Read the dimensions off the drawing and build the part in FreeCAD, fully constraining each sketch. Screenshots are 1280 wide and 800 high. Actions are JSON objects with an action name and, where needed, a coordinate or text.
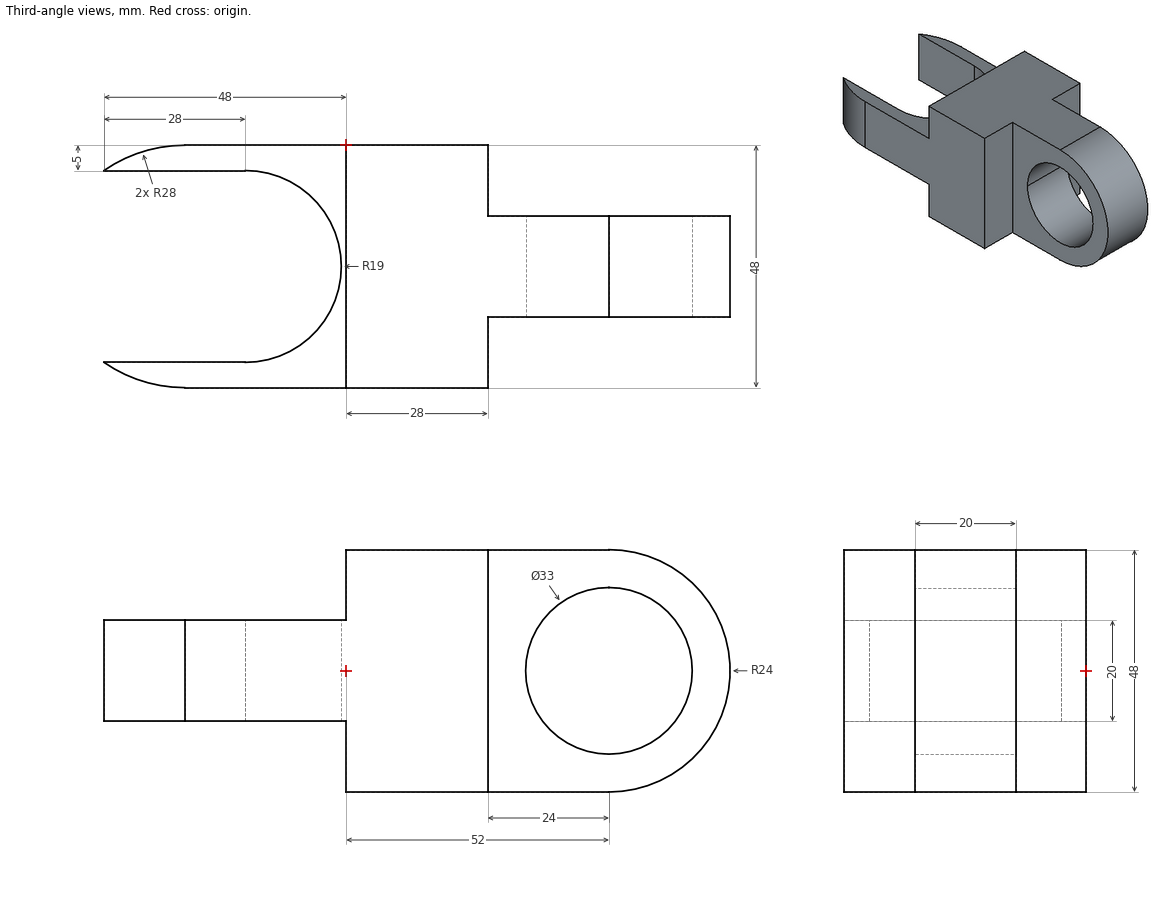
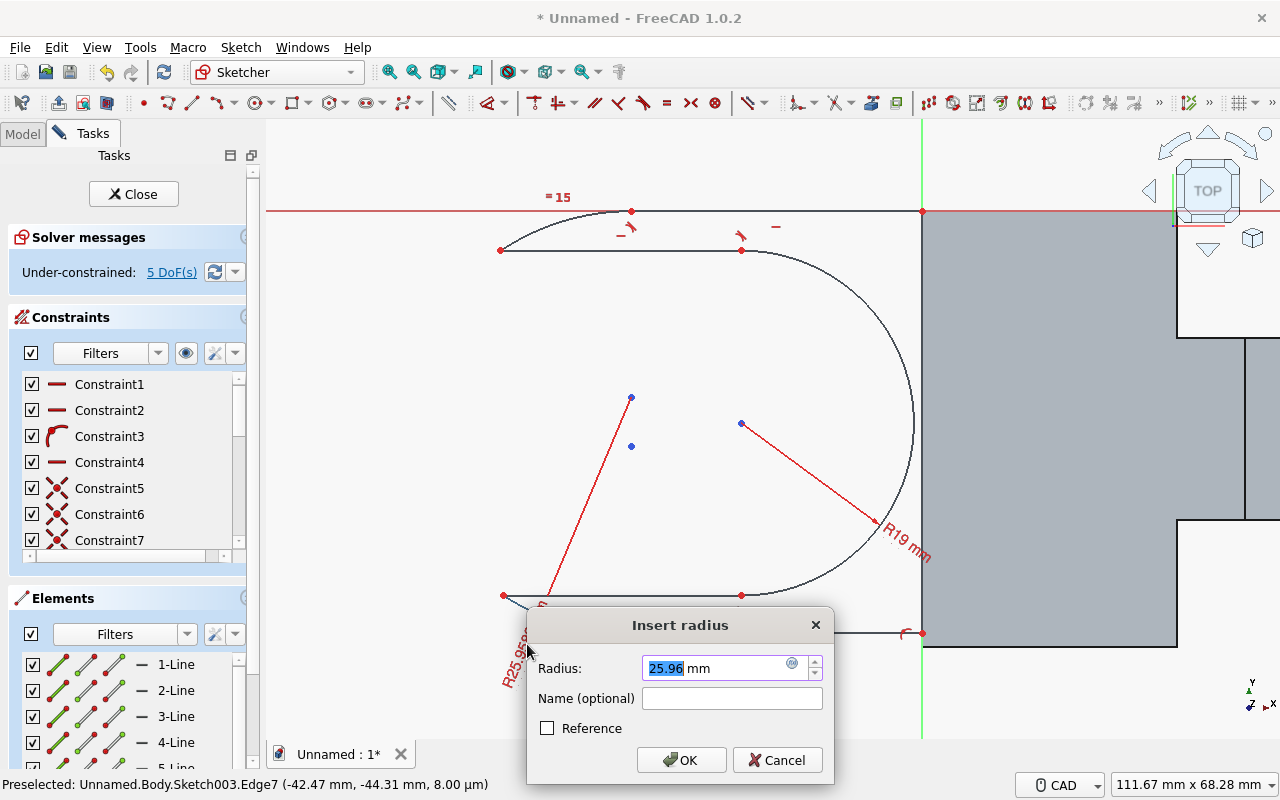
{"action": "type", "text": "28"}
{"action": "key", "text": "Return"}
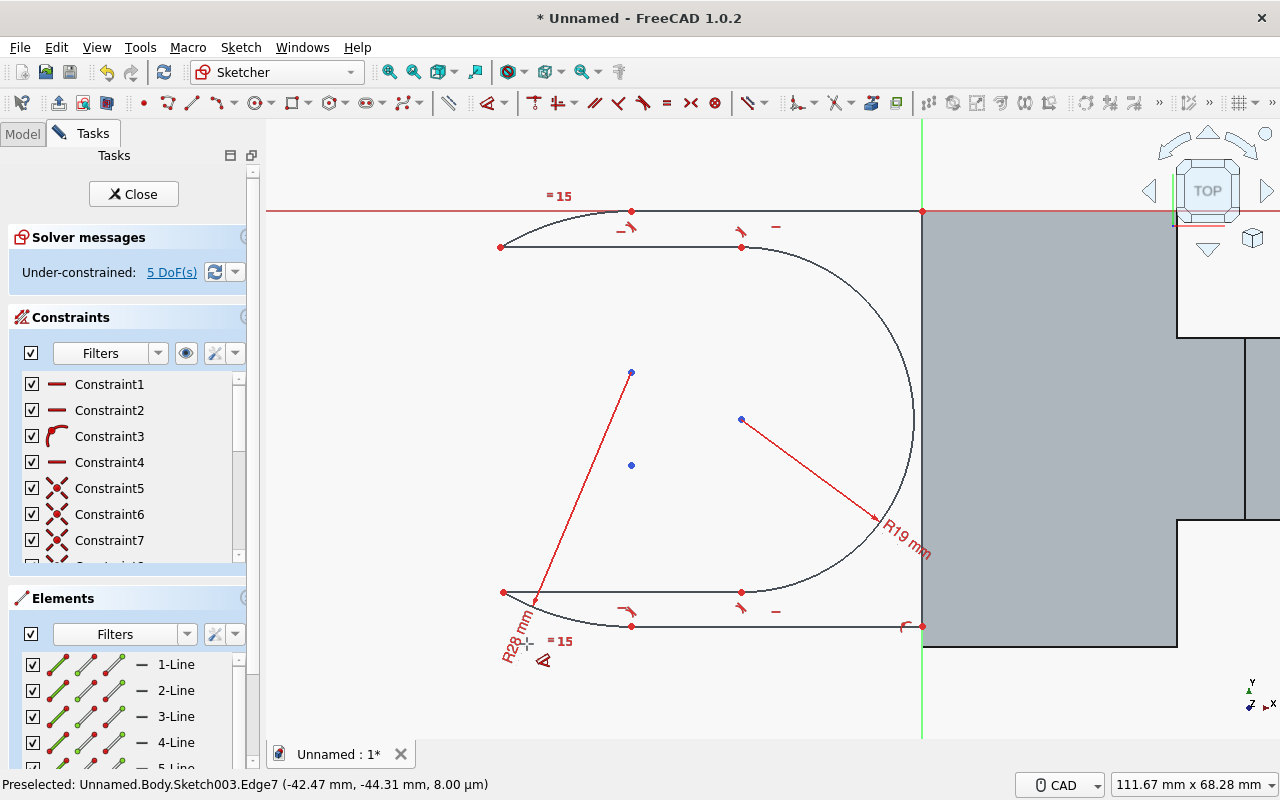
{"action": "left_click", "coordinate": [573, 247]}
{"action": "left_click", "coordinate": [621, 281]}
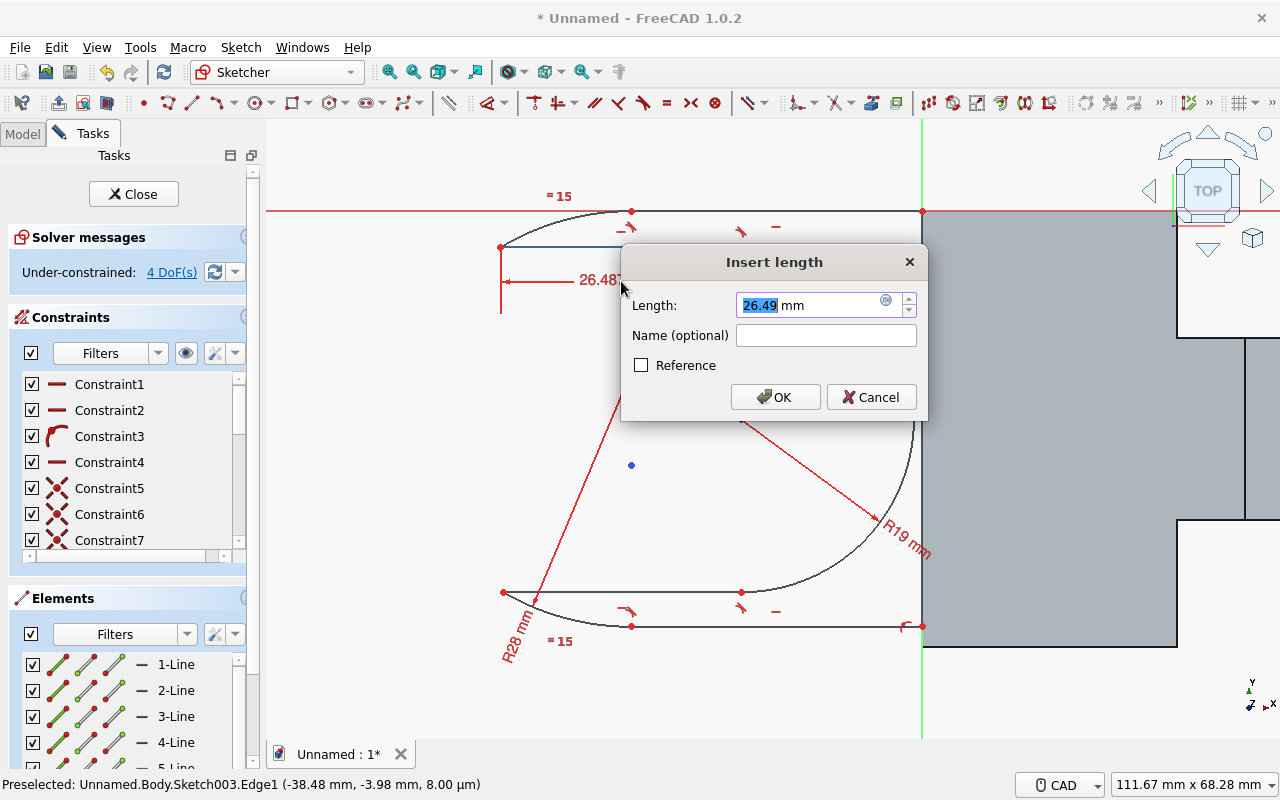
{"action": "type", "text": "28"}
{"action": "key", "text": "Return"}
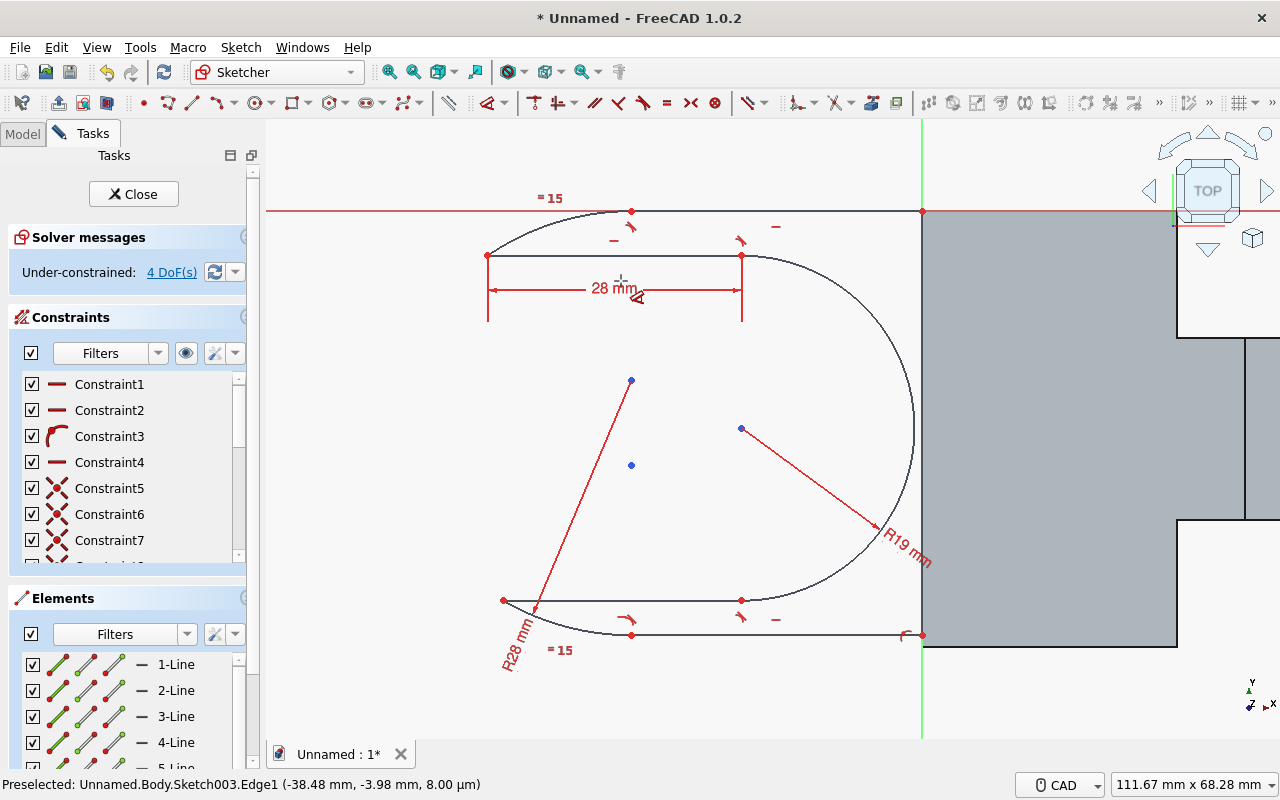
{"action": "left_click", "coordinate": [670, 601]}
{"action": "left_click", "coordinate": [623, 567]}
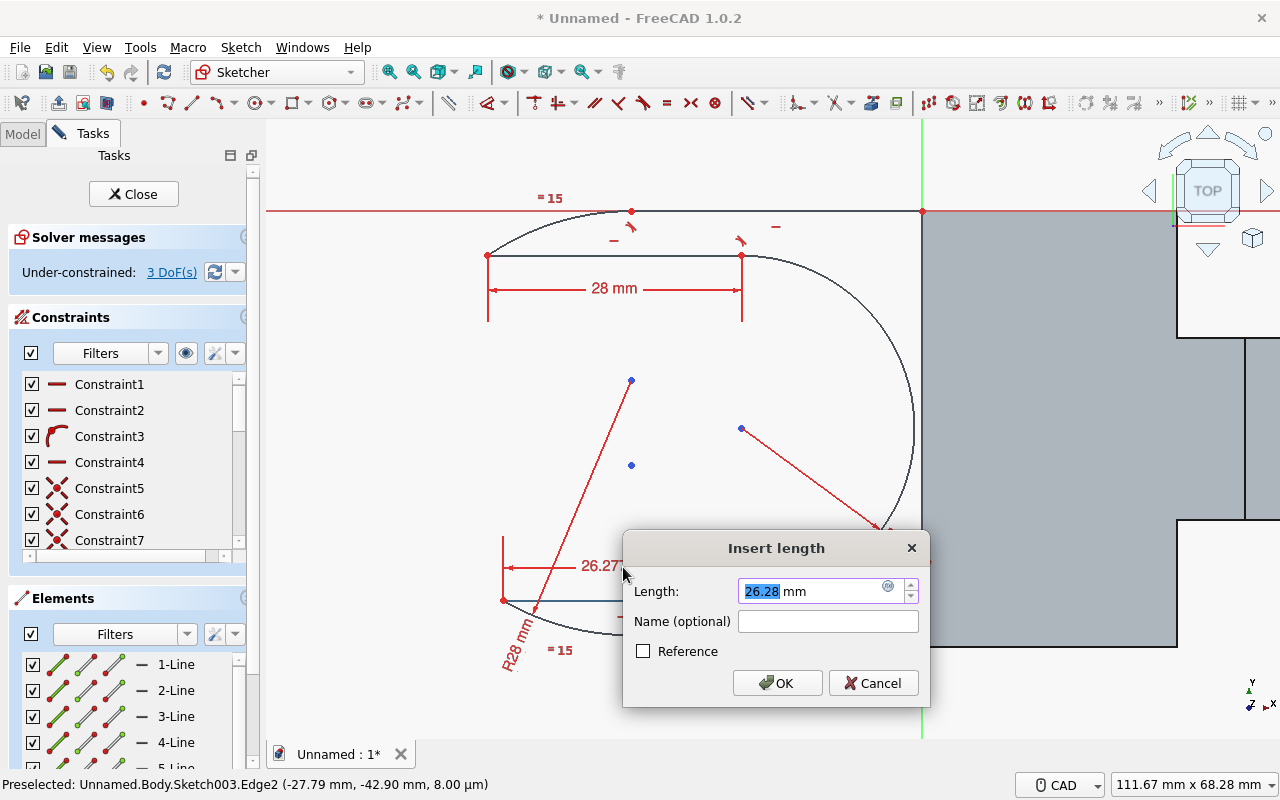
{"action": "type", "text": "28"}
{"action": "key", "text": "Return"}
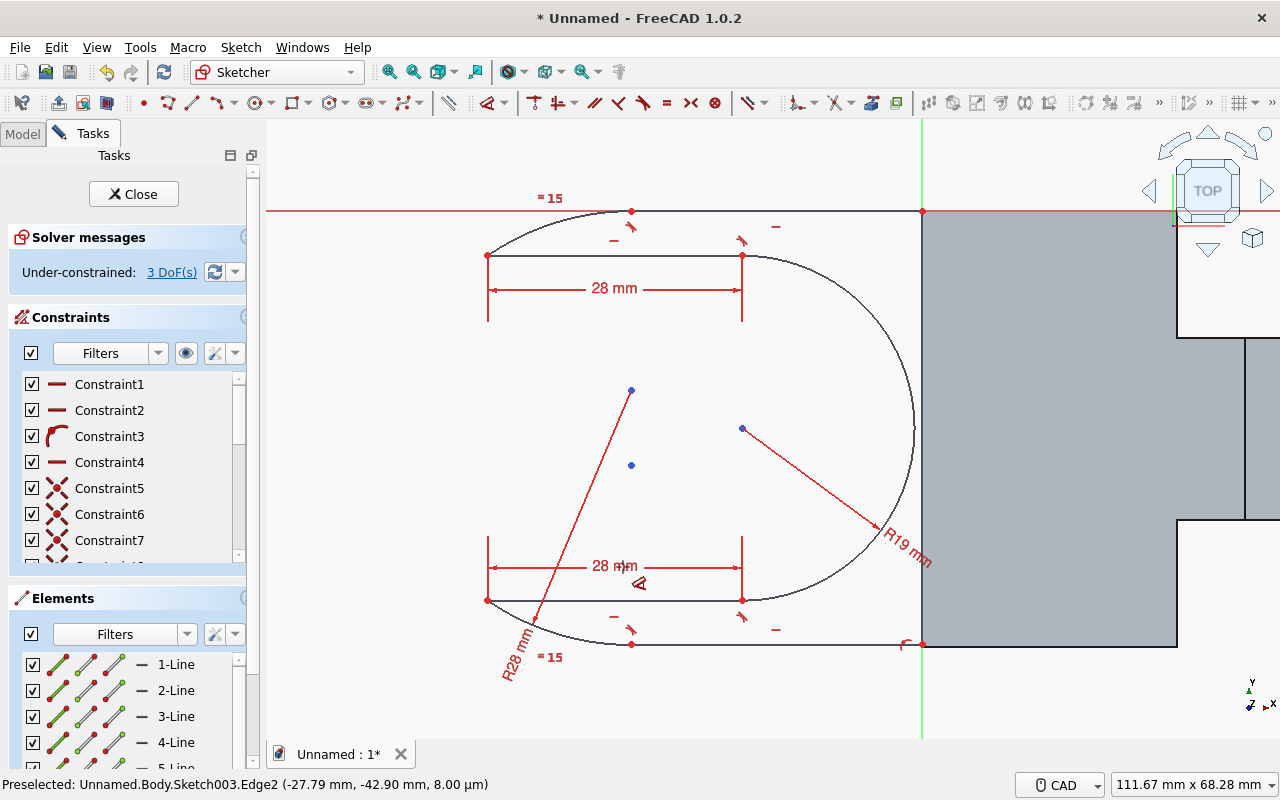
{"action": "left_click", "coordinate": [922, 515]}
{"action": "left_click", "coordinate": [956, 428]}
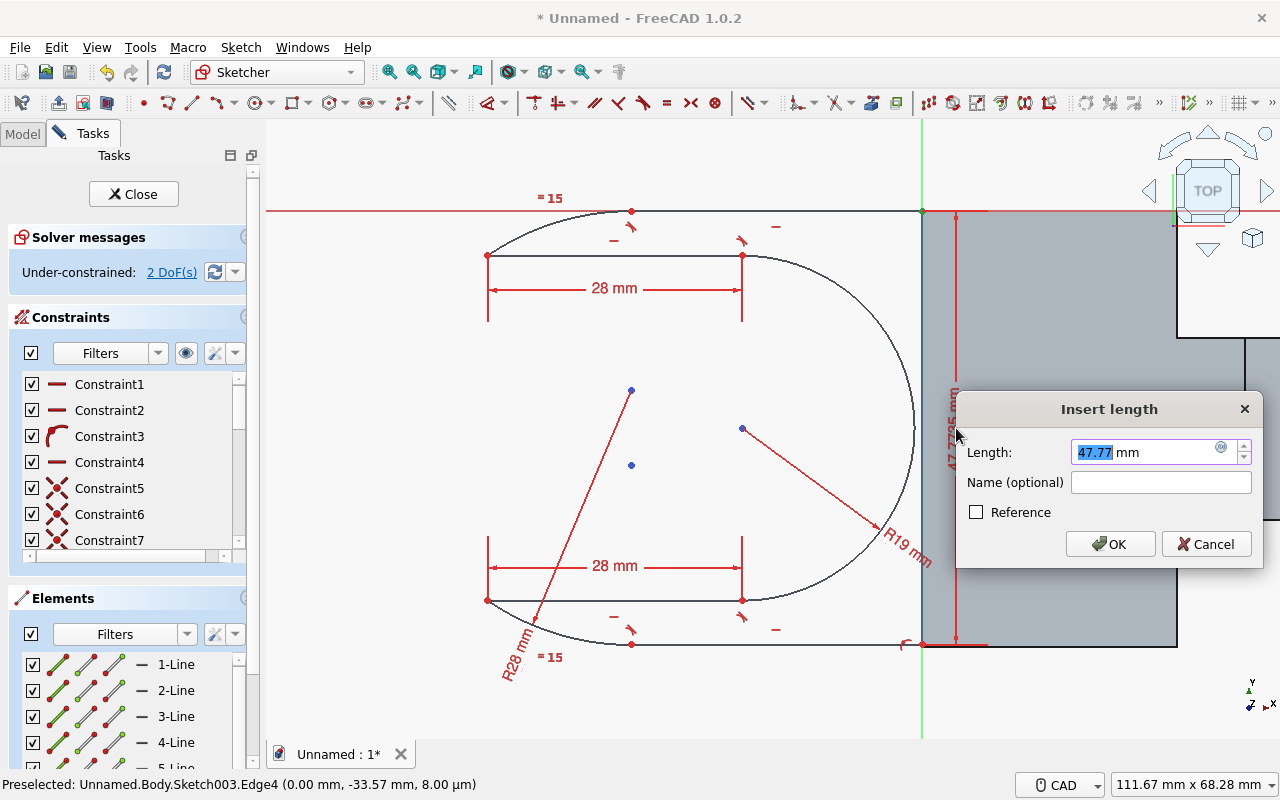
{"action": "type", "text": "48"}
{"action": "key", "text": "Return"}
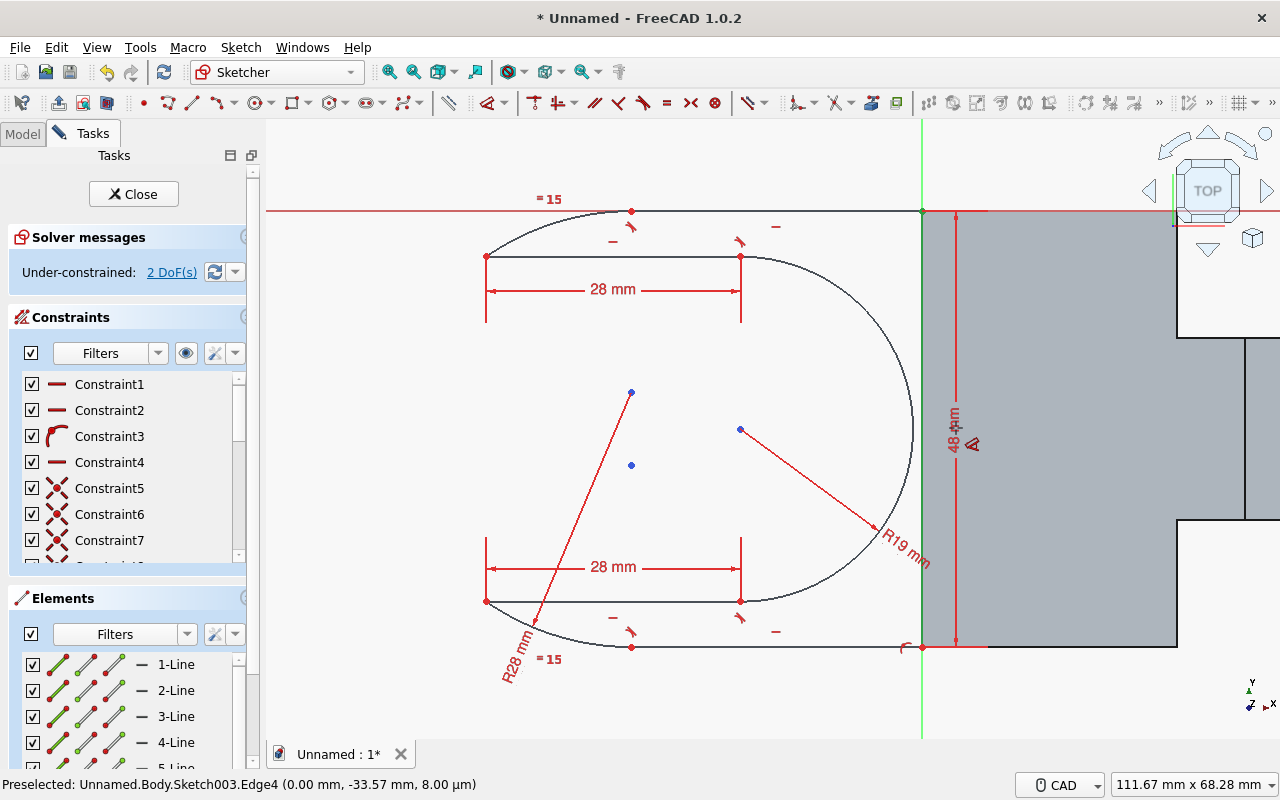
{"action": "left_click", "coordinate": [486, 257]}
{"action": "left_click", "coordinate": [452, 234]}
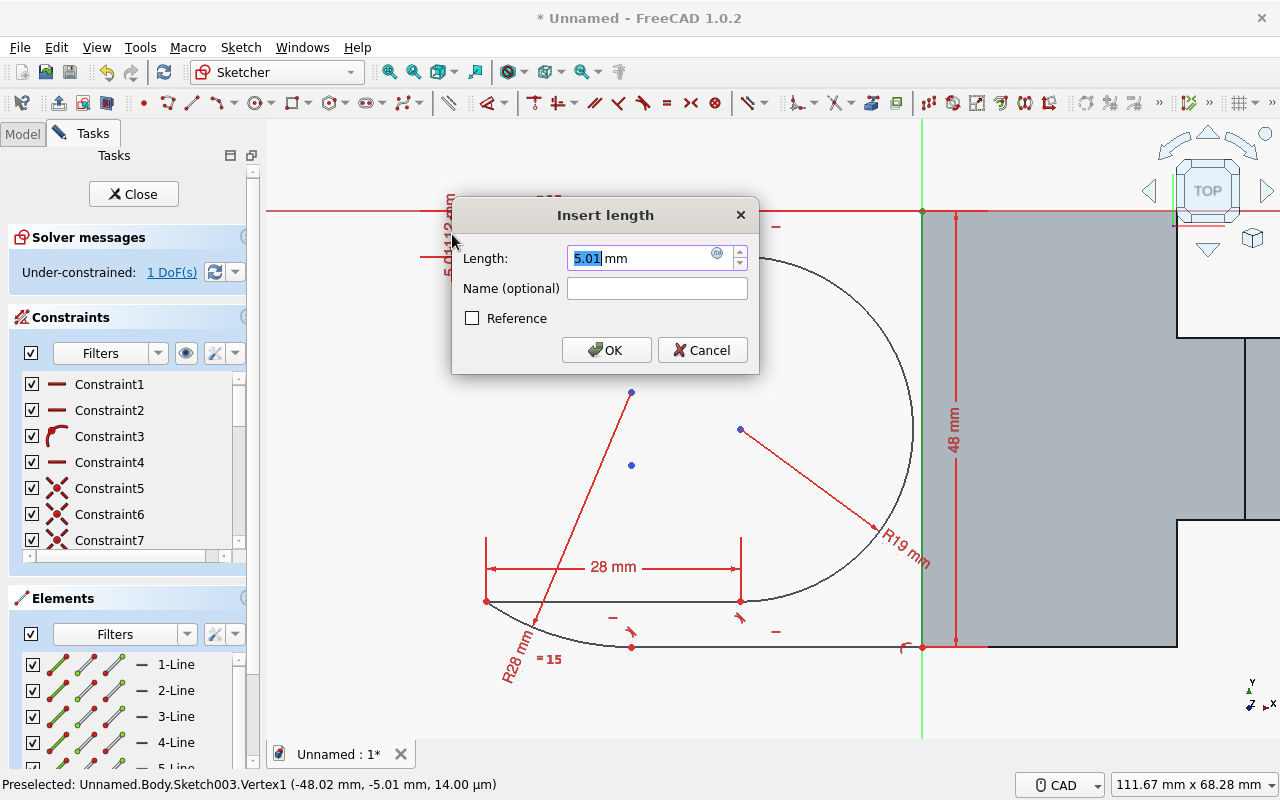
{"action": "type", "text": "5"}
{"action": "key", "text": "Return"}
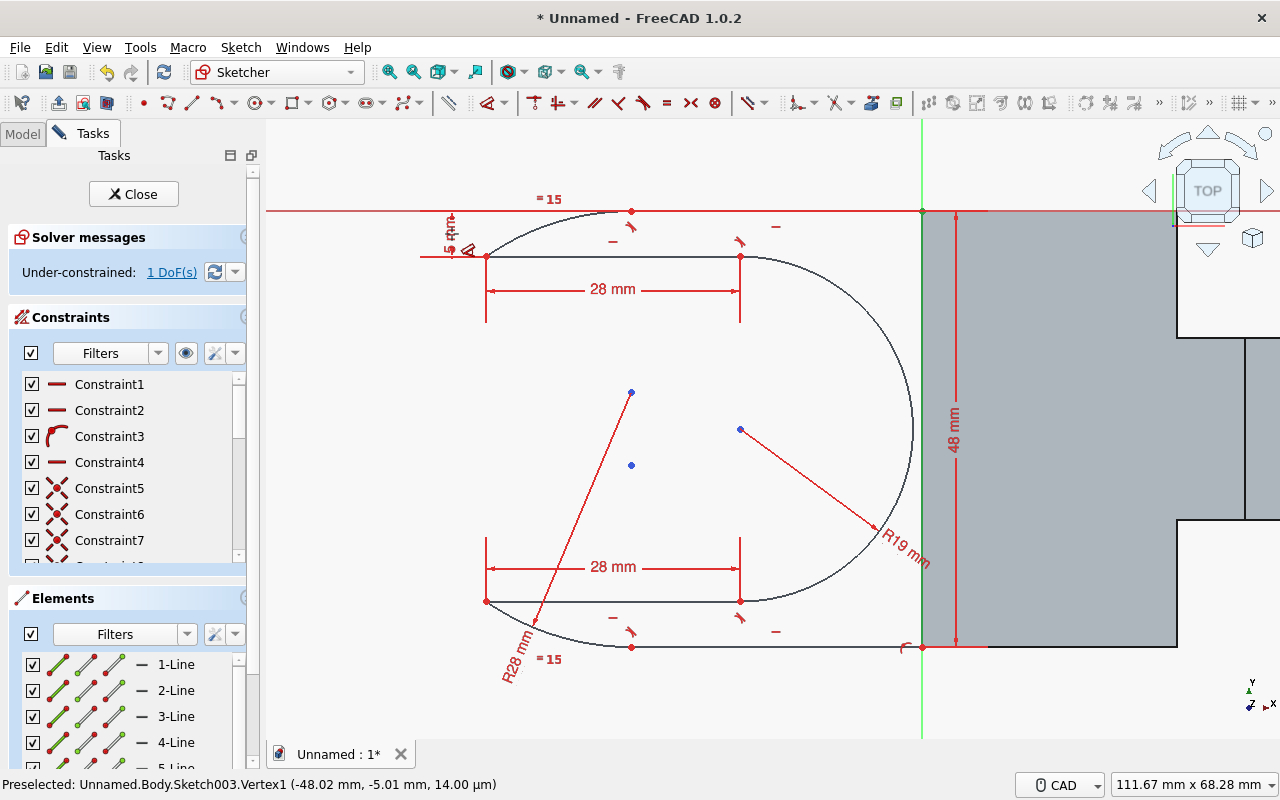
{"action": "left_click", "coordinate": [486, 257]}
{"action": "left_click", "coordinate": [704, 177]}